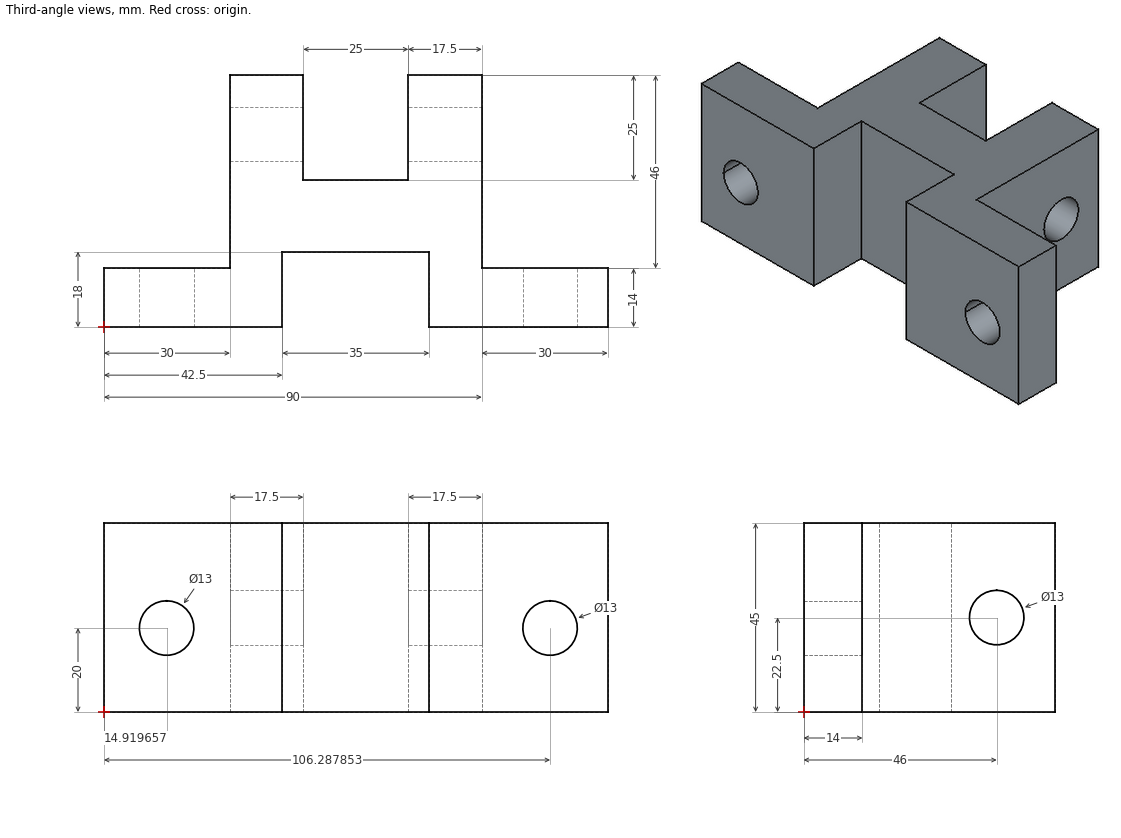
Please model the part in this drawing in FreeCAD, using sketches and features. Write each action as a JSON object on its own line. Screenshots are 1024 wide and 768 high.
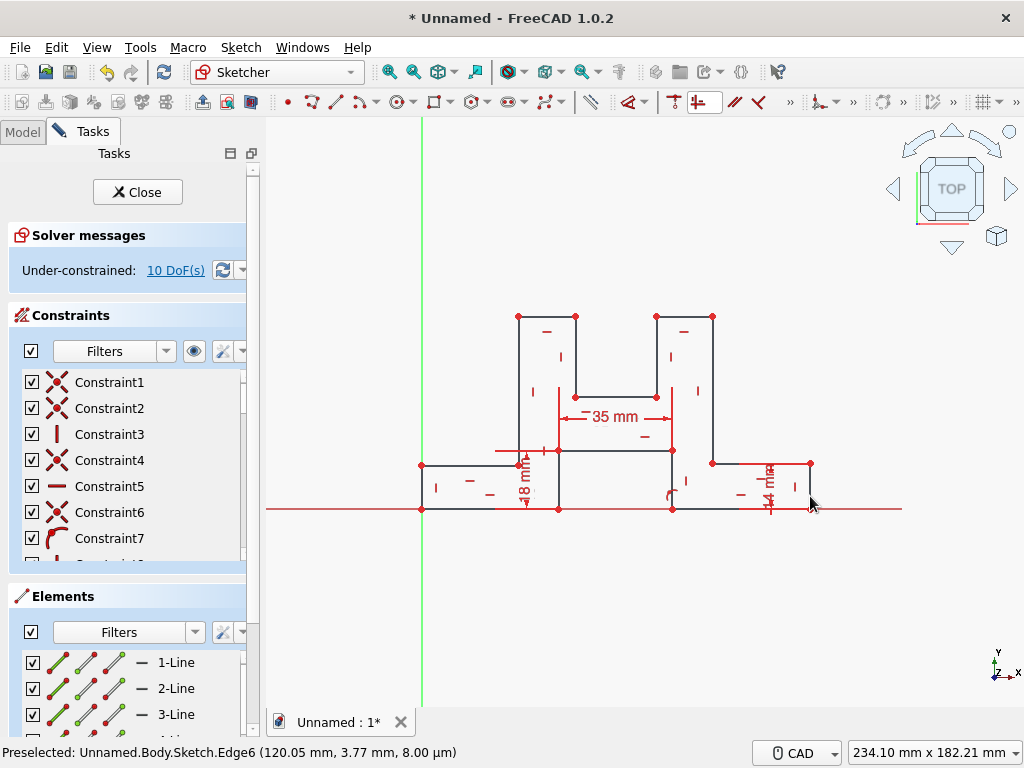
{"action": "left_click", "coordinate": [781, 464]}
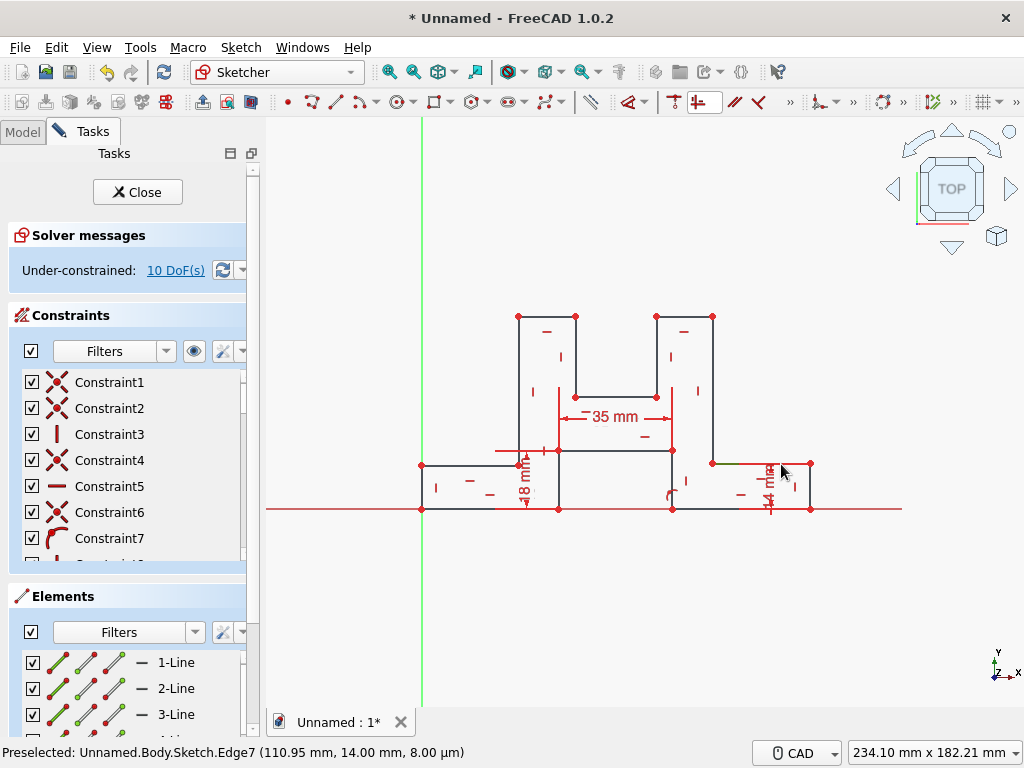
{"action": "key", "text": "l"}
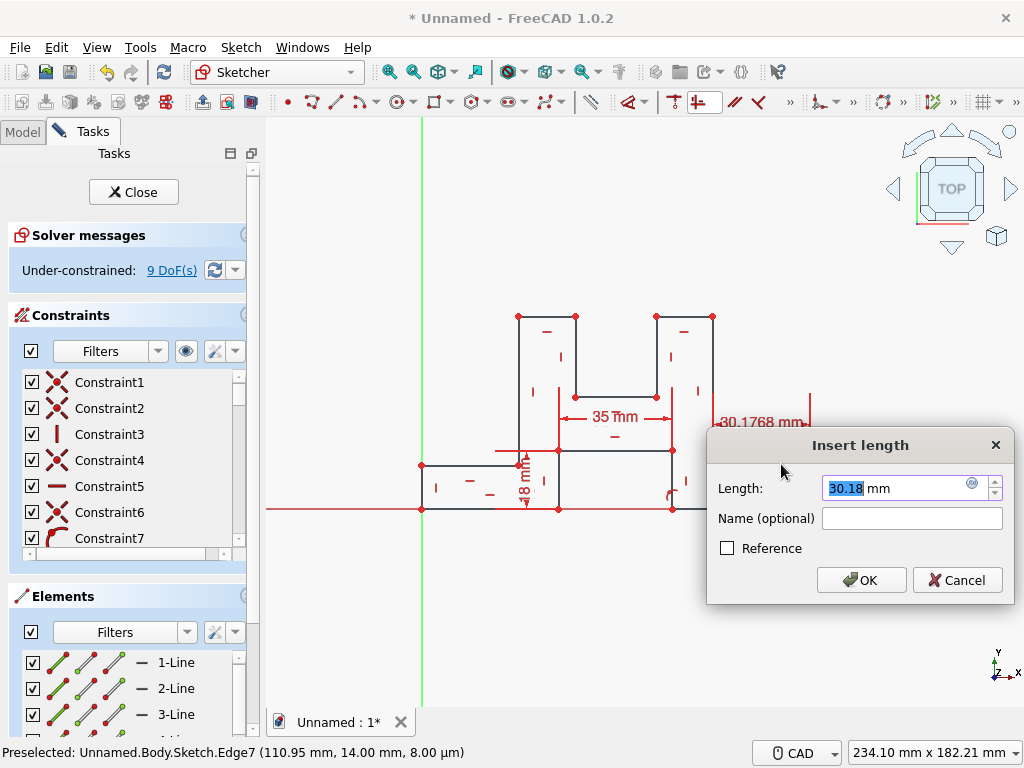
{"action": "type", "text": "30"}
{"action": "key", "text": "Return"}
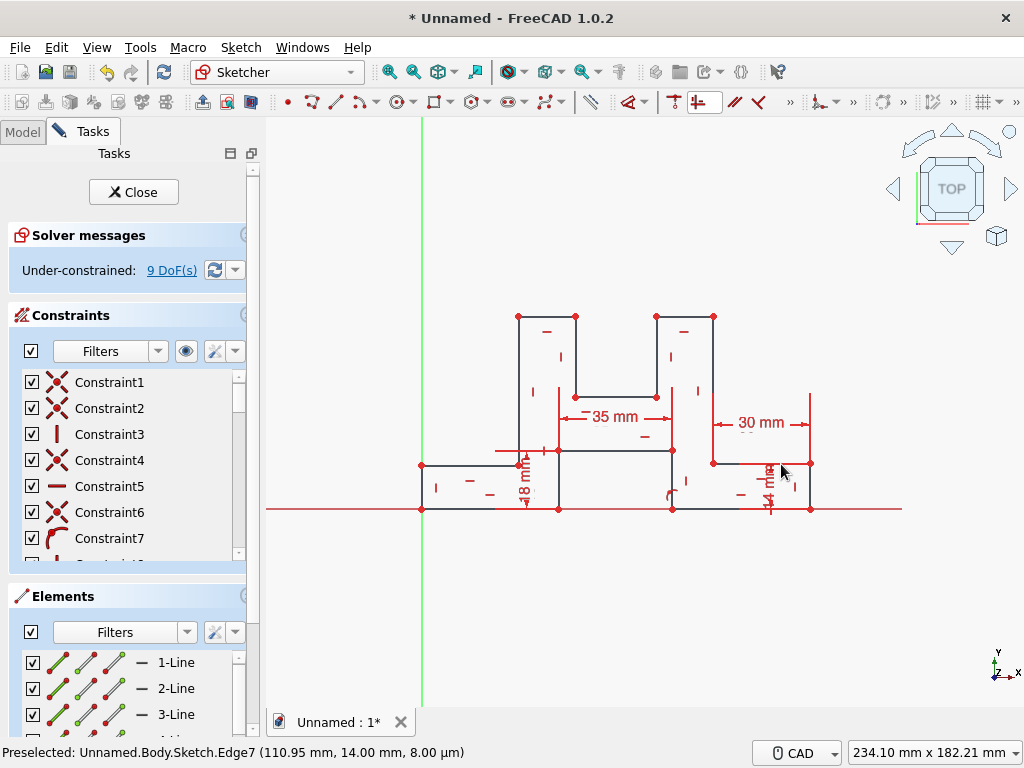
{"action": "left_click", "coordinate": [713, 420]}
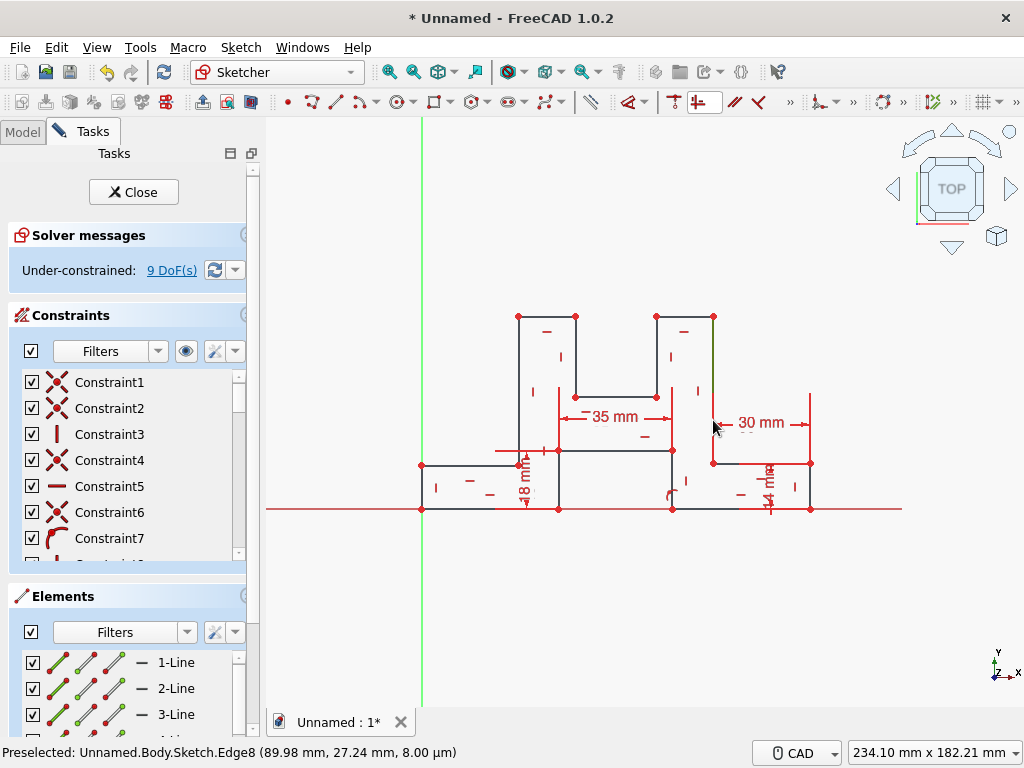
{"action": "key", "text": "i"}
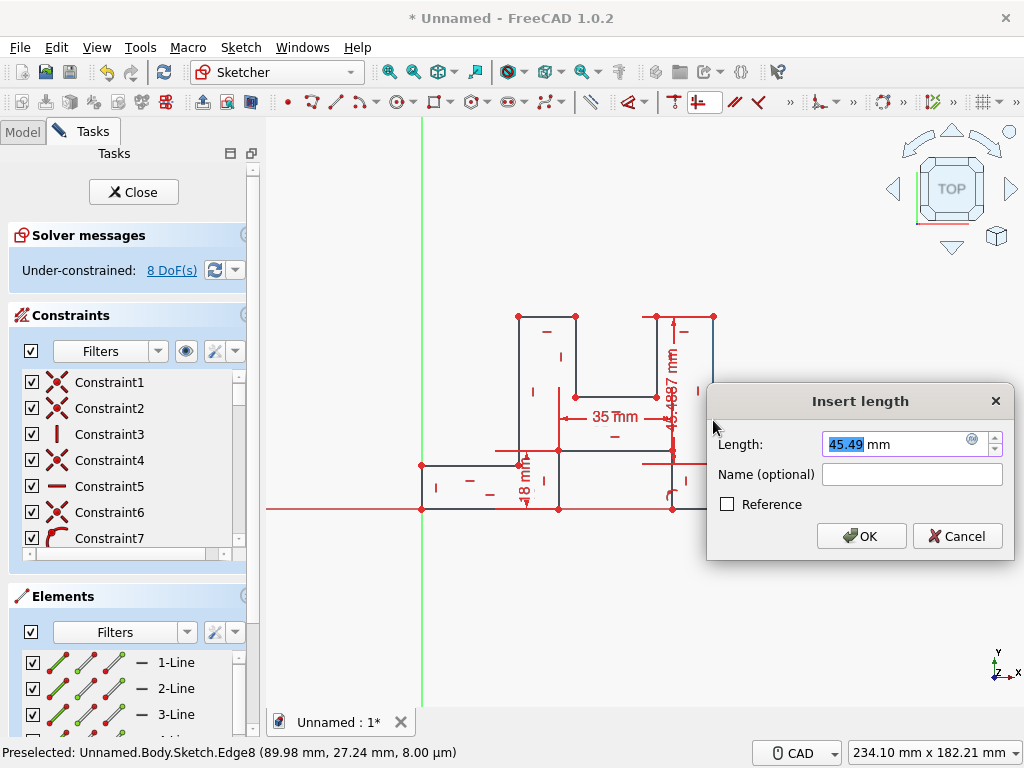
{"action": "type", "text": "46"}
{"action": "key", "text": "Return"}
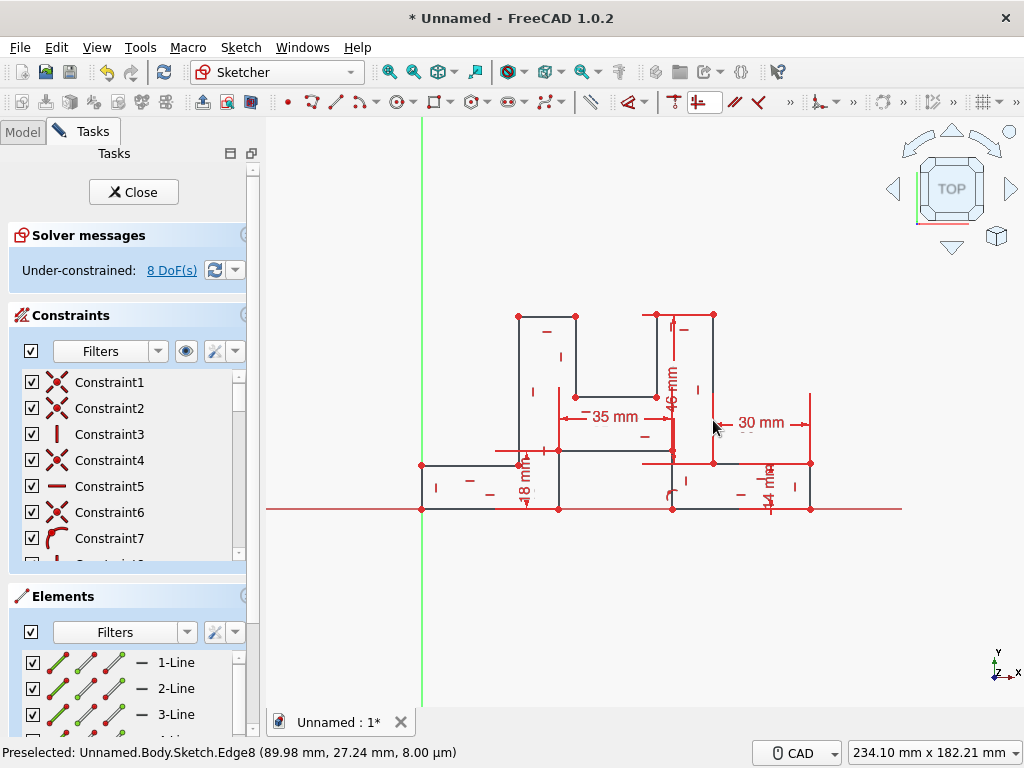
{"action": "left_click", "coordinate": [657, 340]}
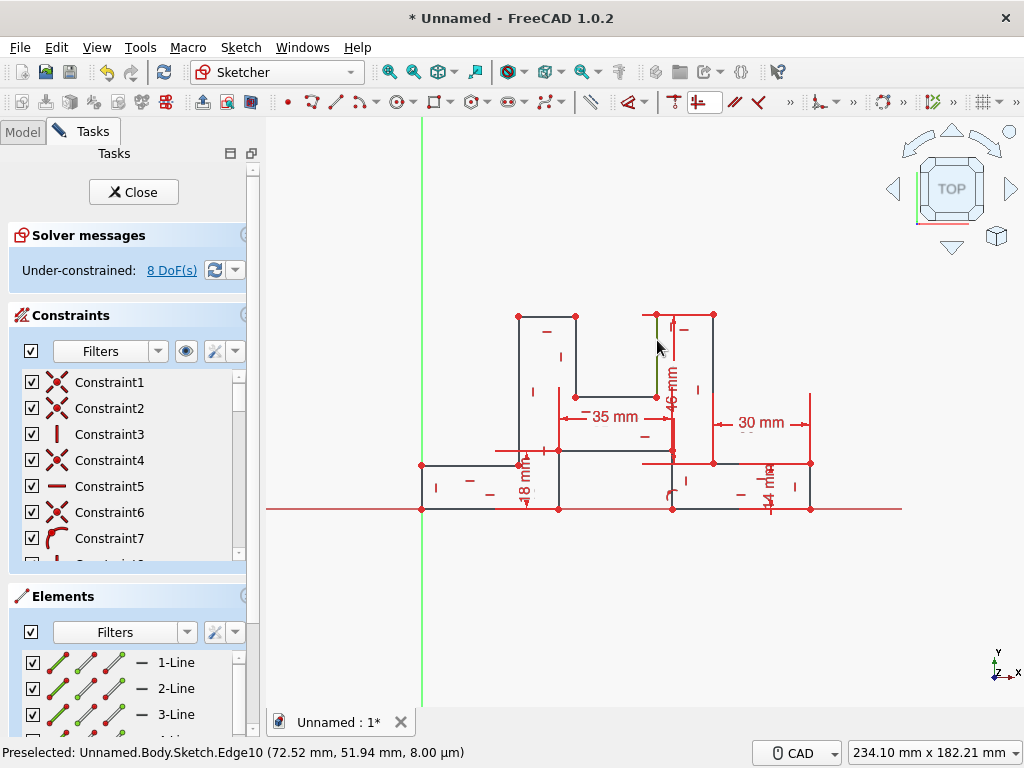
{"action": "key", "text": "i"}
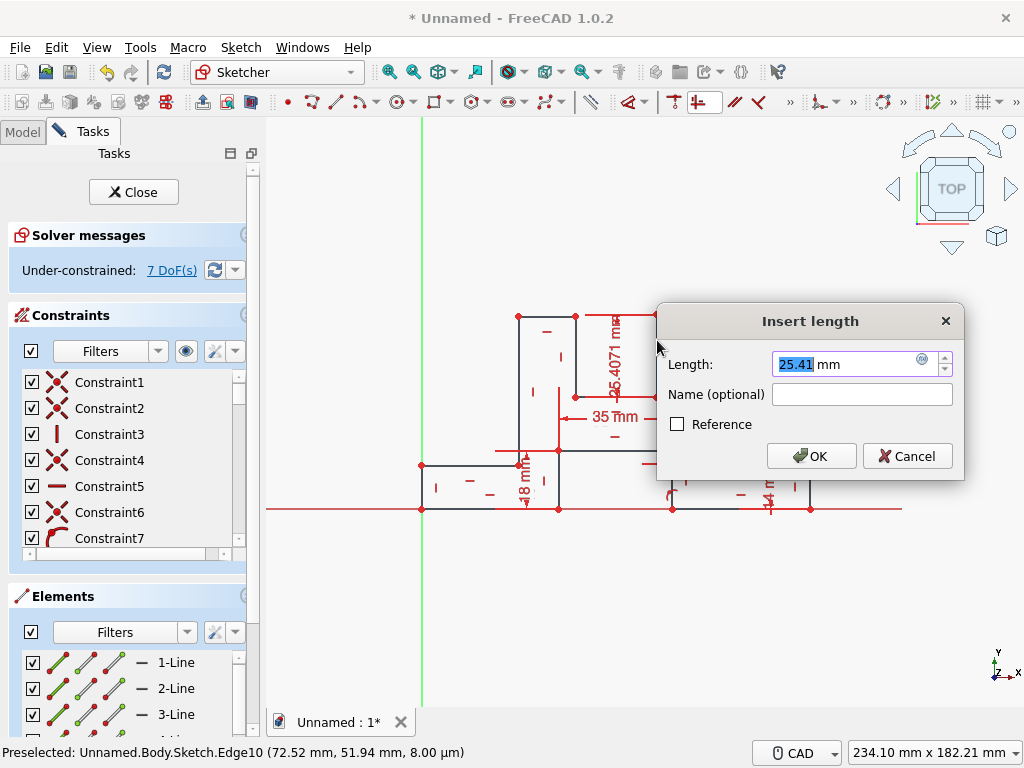
{"action": "type", "text": "25"}
{"action": "key", "text": "Return"}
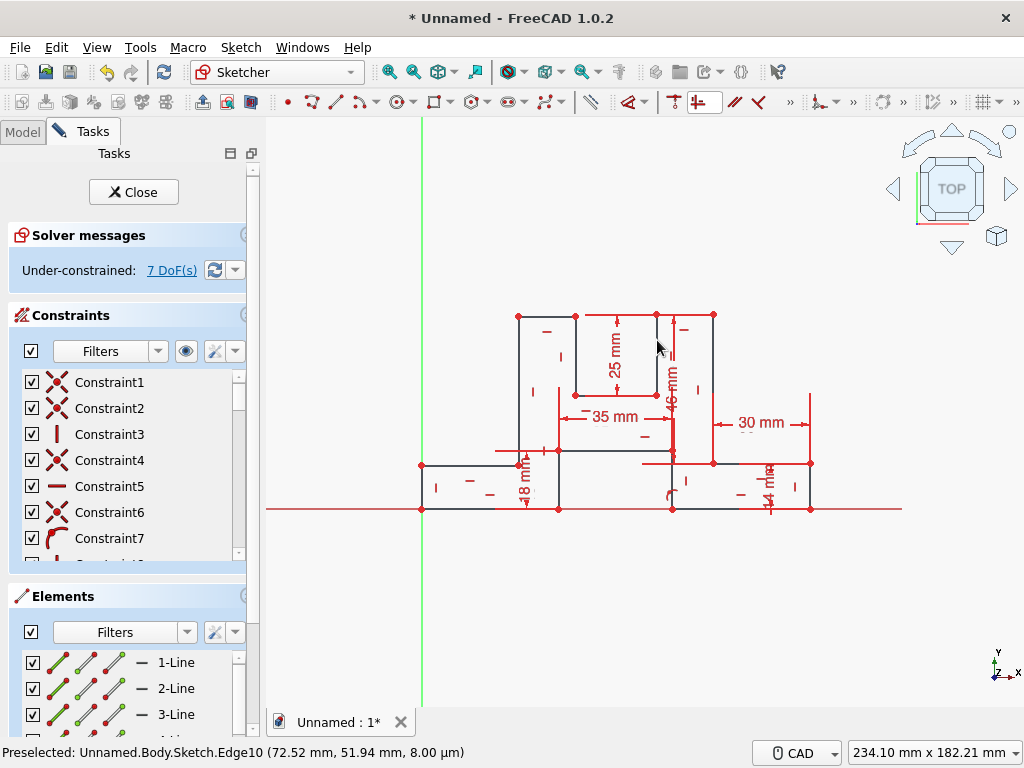
{"action": "left_click", "coordinate": [632, 396]}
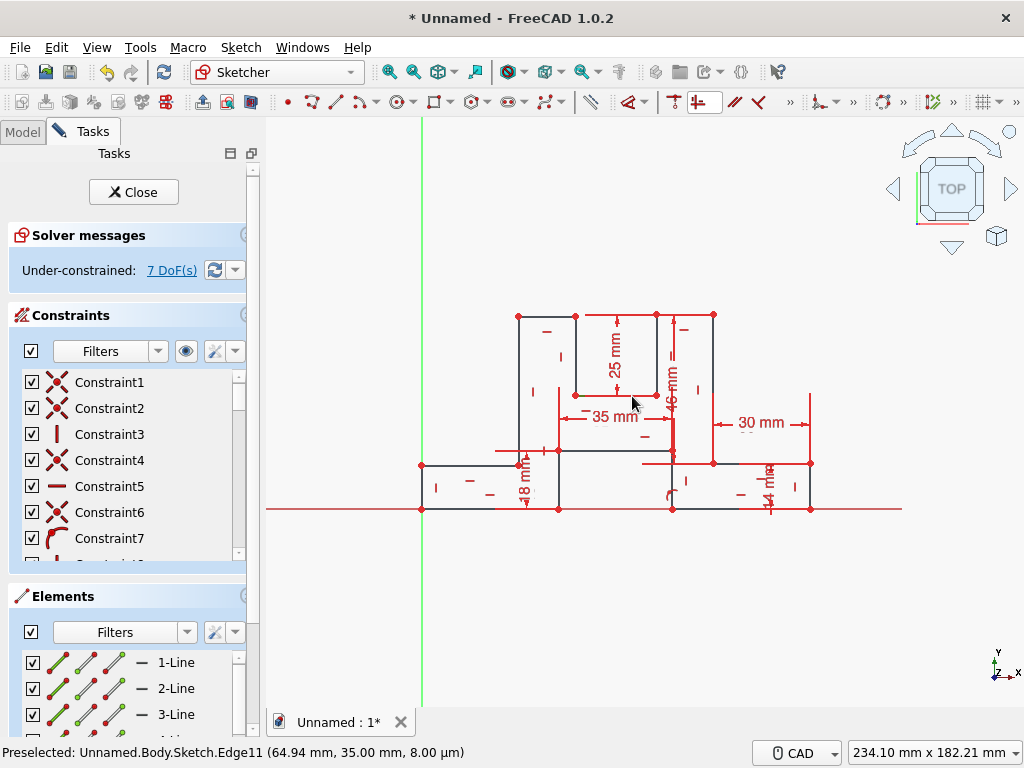
{"action": "key", "text": "l"}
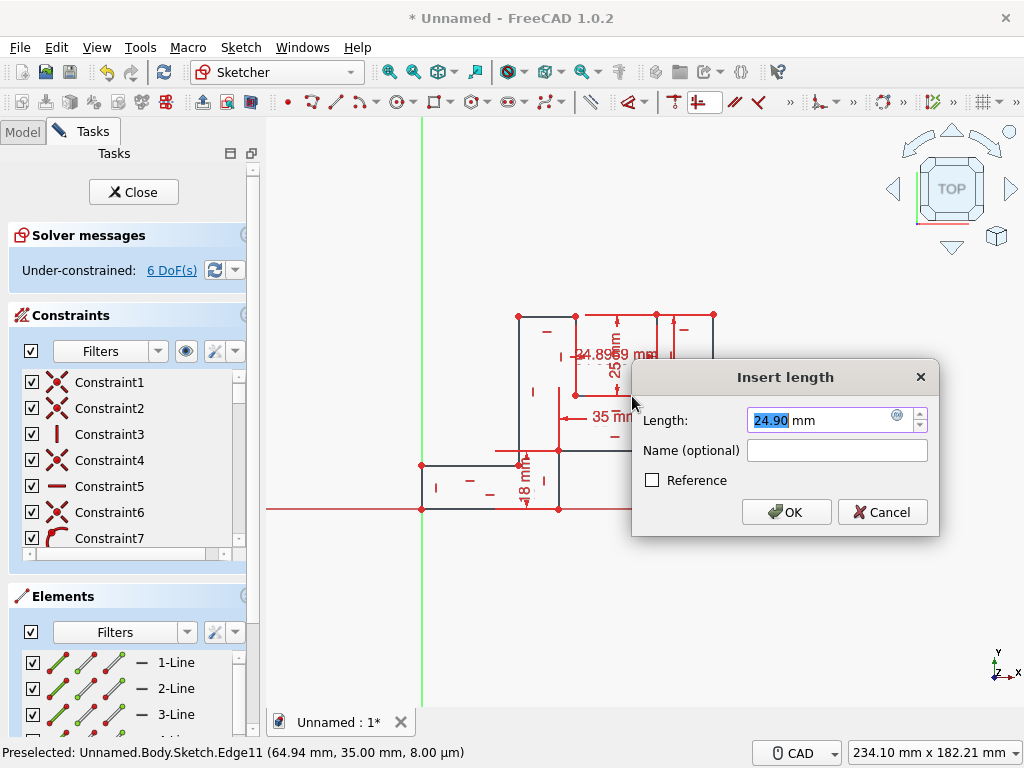
{"action": "type", "text": "25"}
{"action": "key", "text": "Return"}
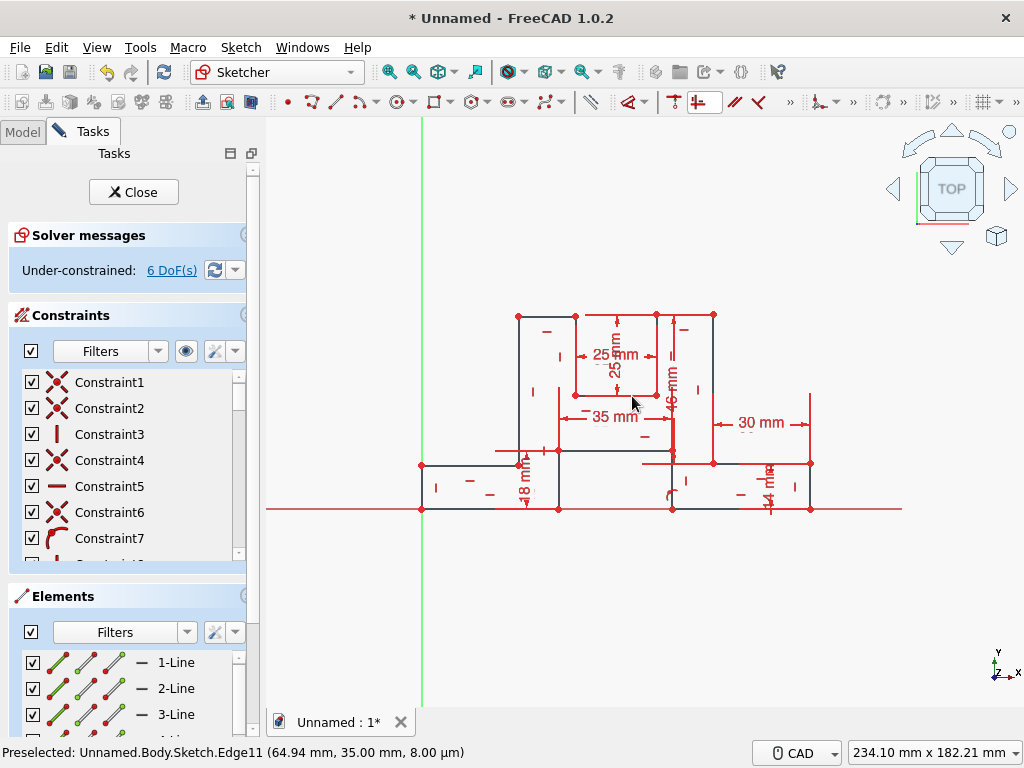
{"action": "left_click", "coordinate": [576, 372]}